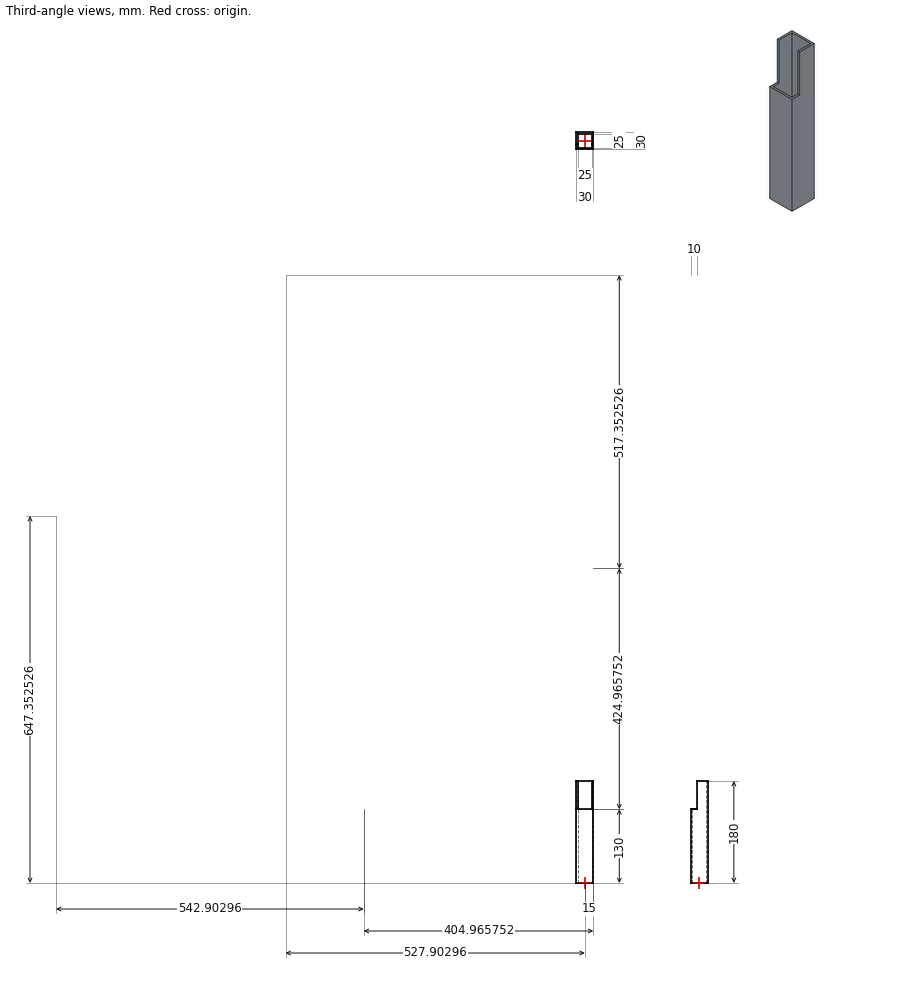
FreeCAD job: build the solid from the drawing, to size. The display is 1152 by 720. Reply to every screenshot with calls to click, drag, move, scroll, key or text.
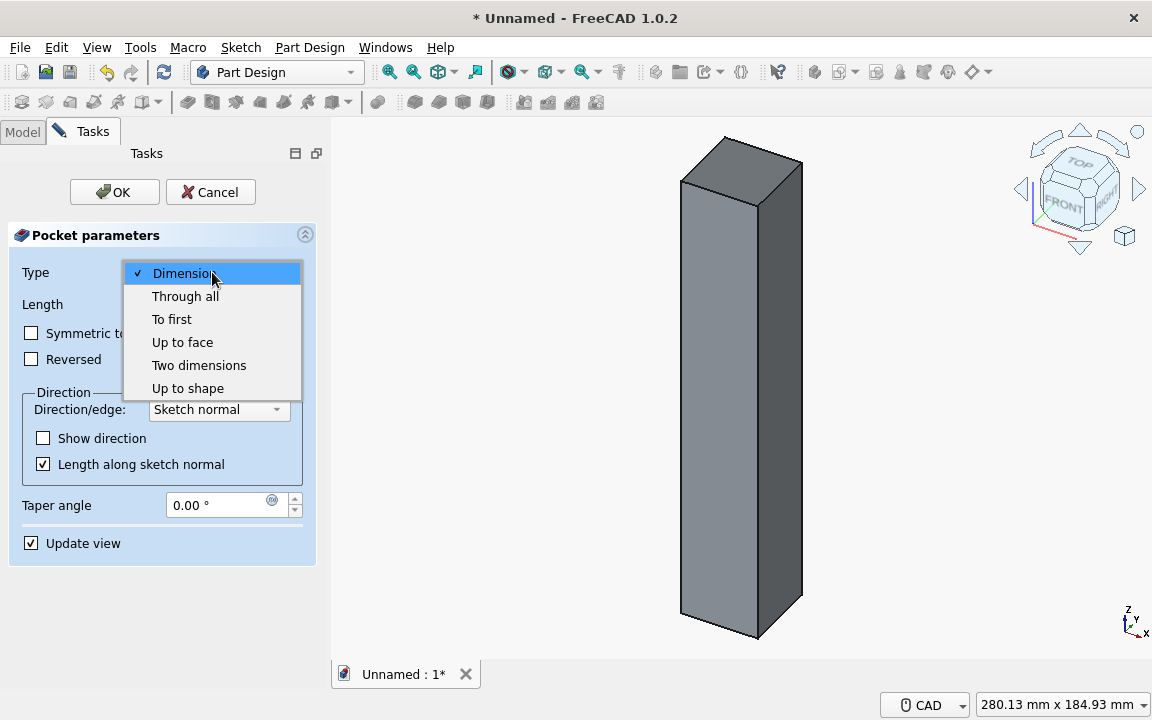
click(212, 296)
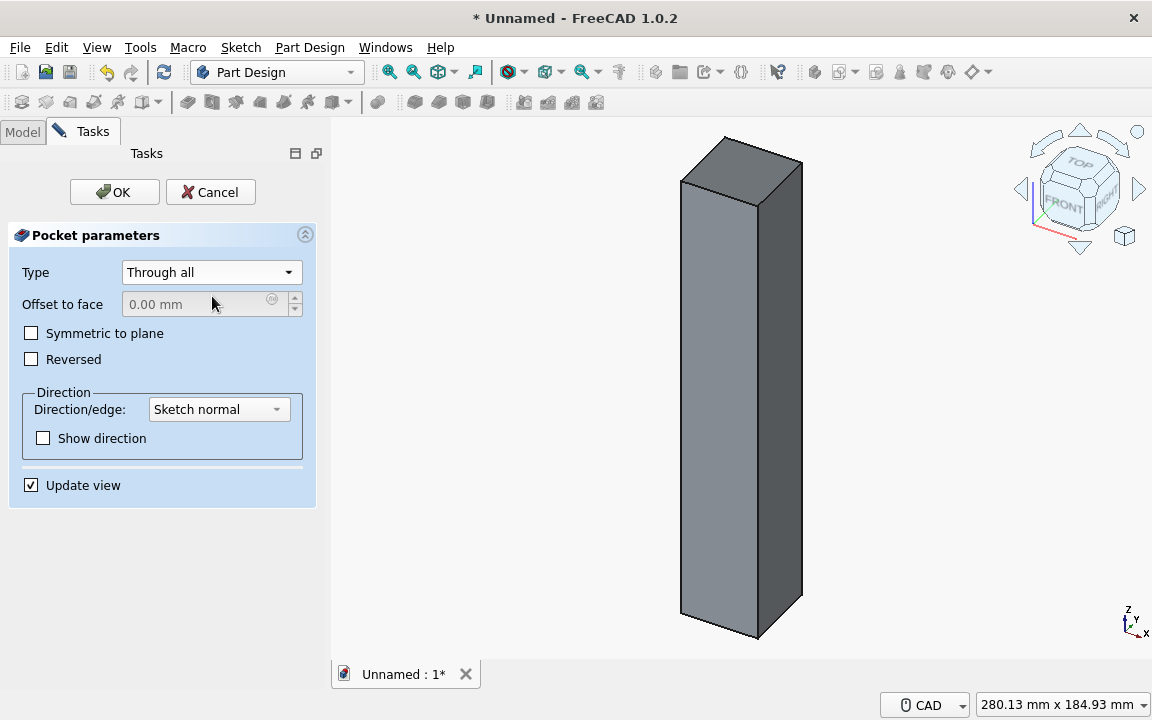
click(30, 359)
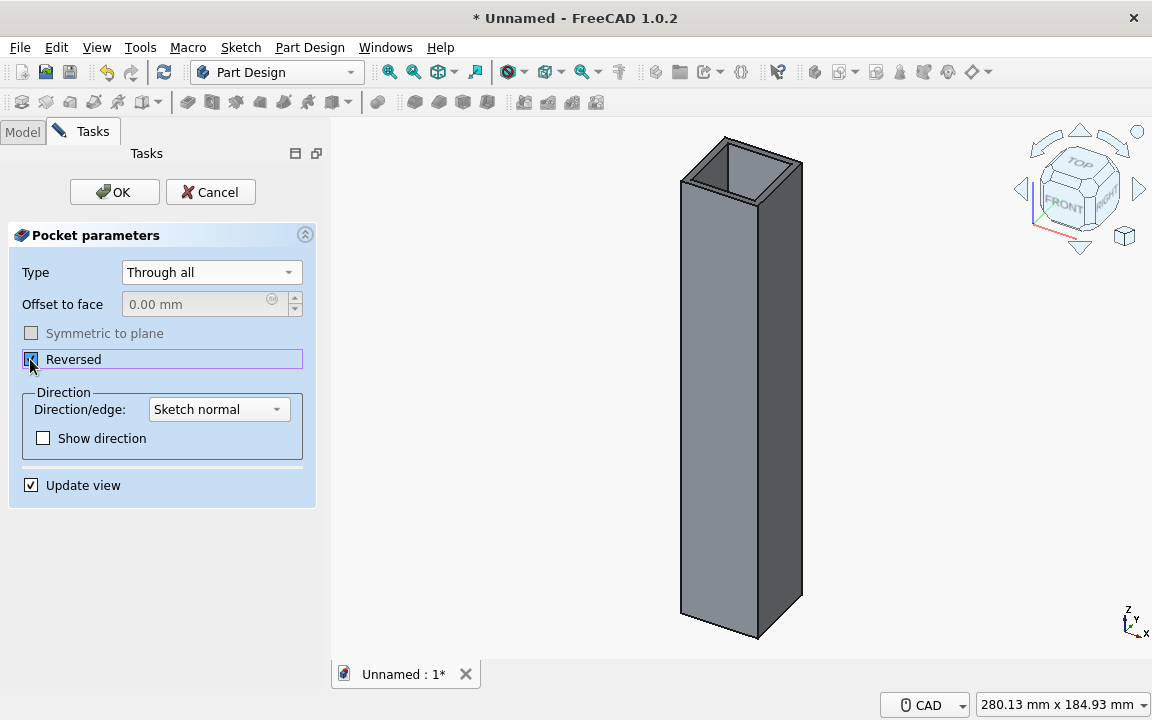
click(115, 192)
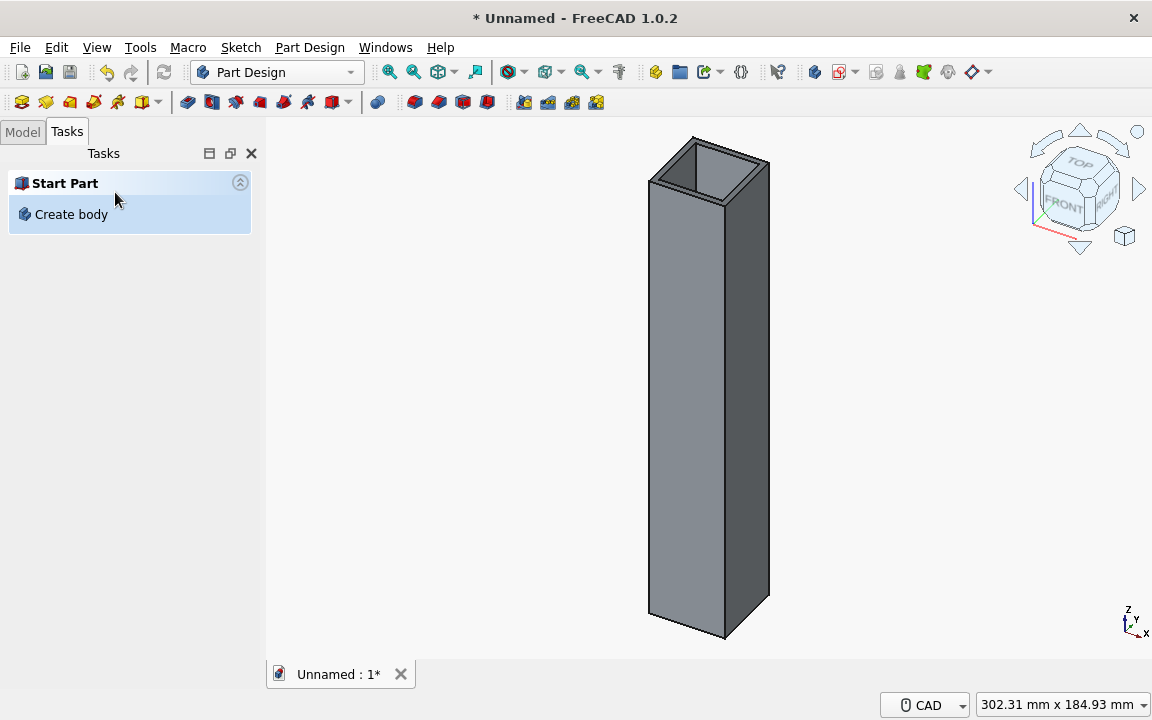
click(687, 285)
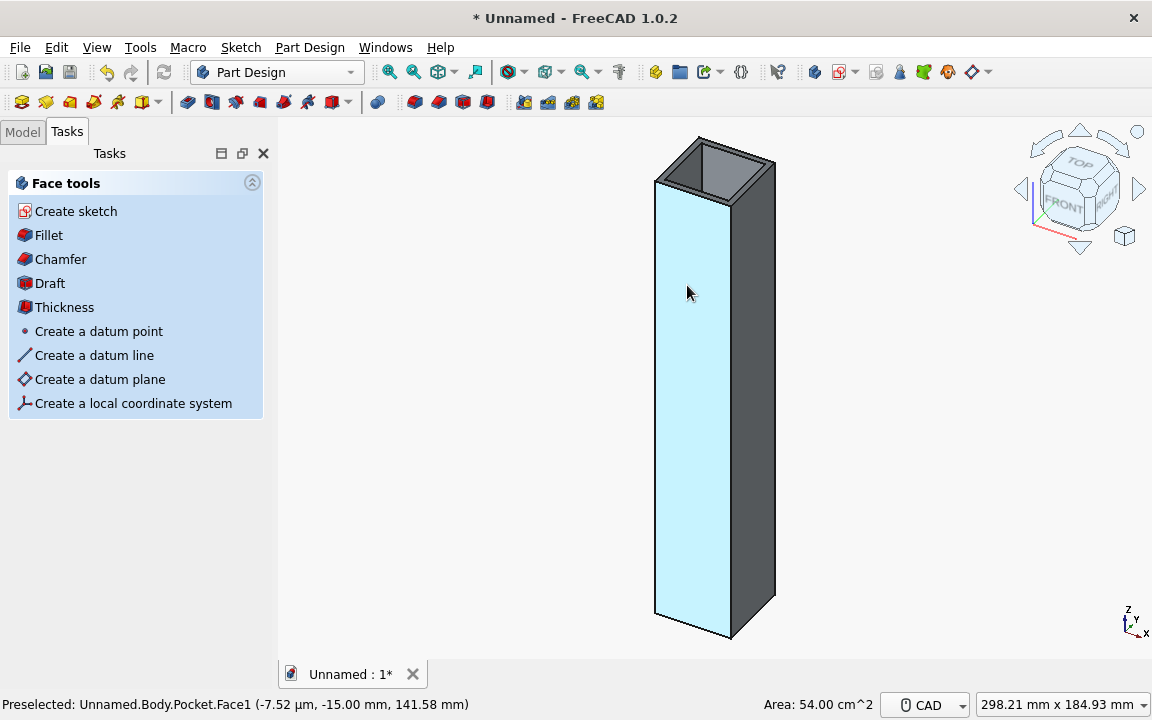
click(840, 72)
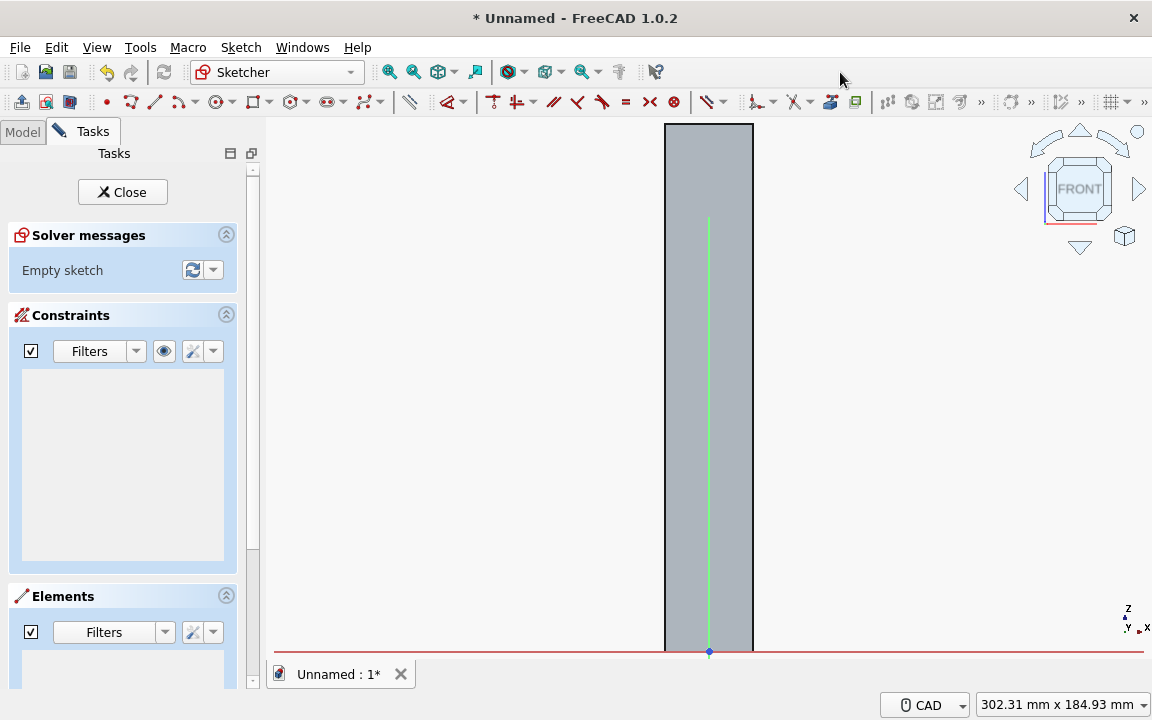
scroll(800, 551, down, 11)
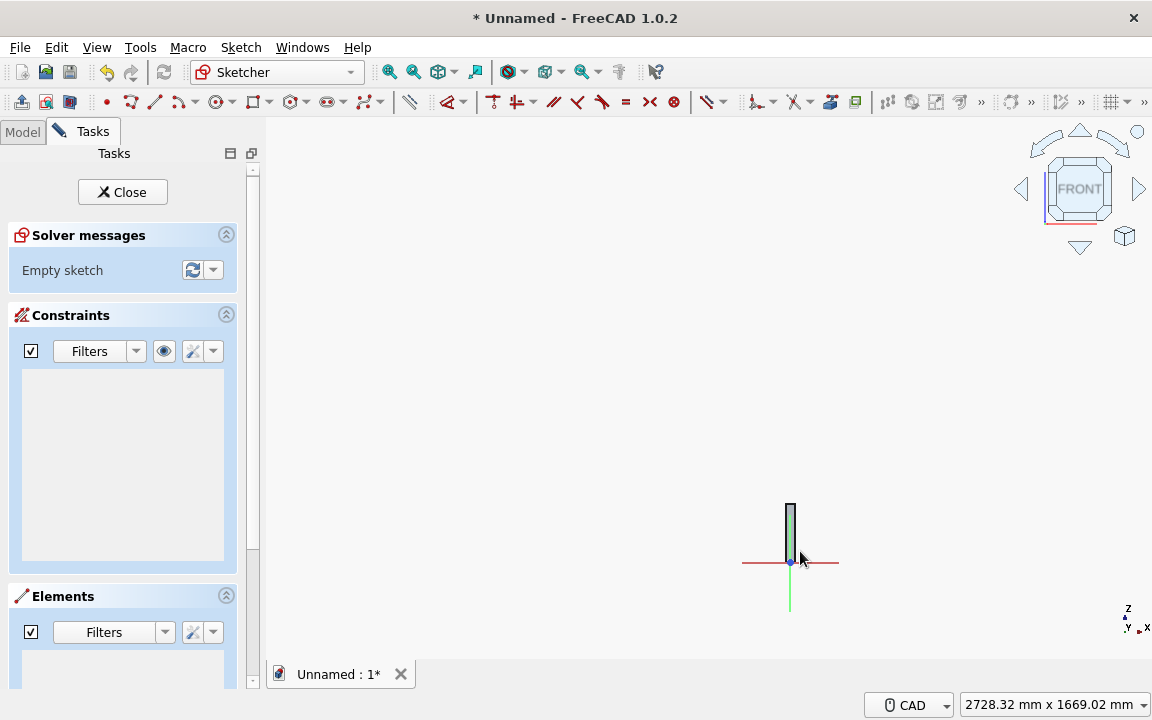
key(g)
key(m)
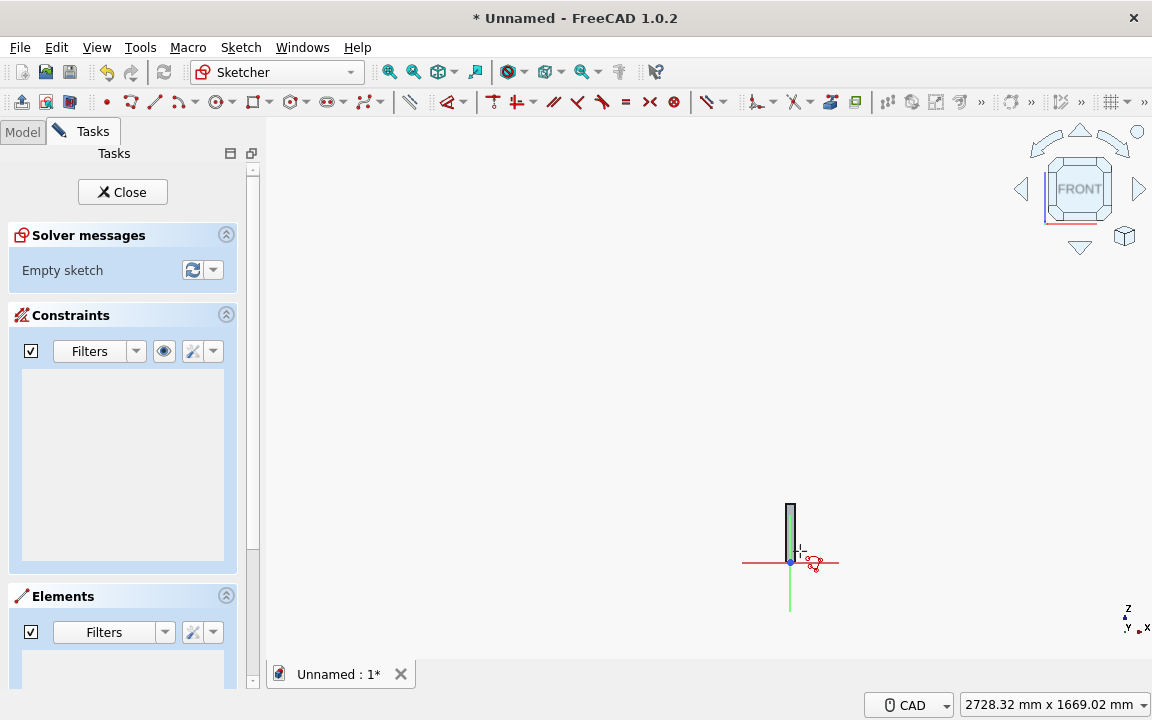
scroll(795, 521, up, 6)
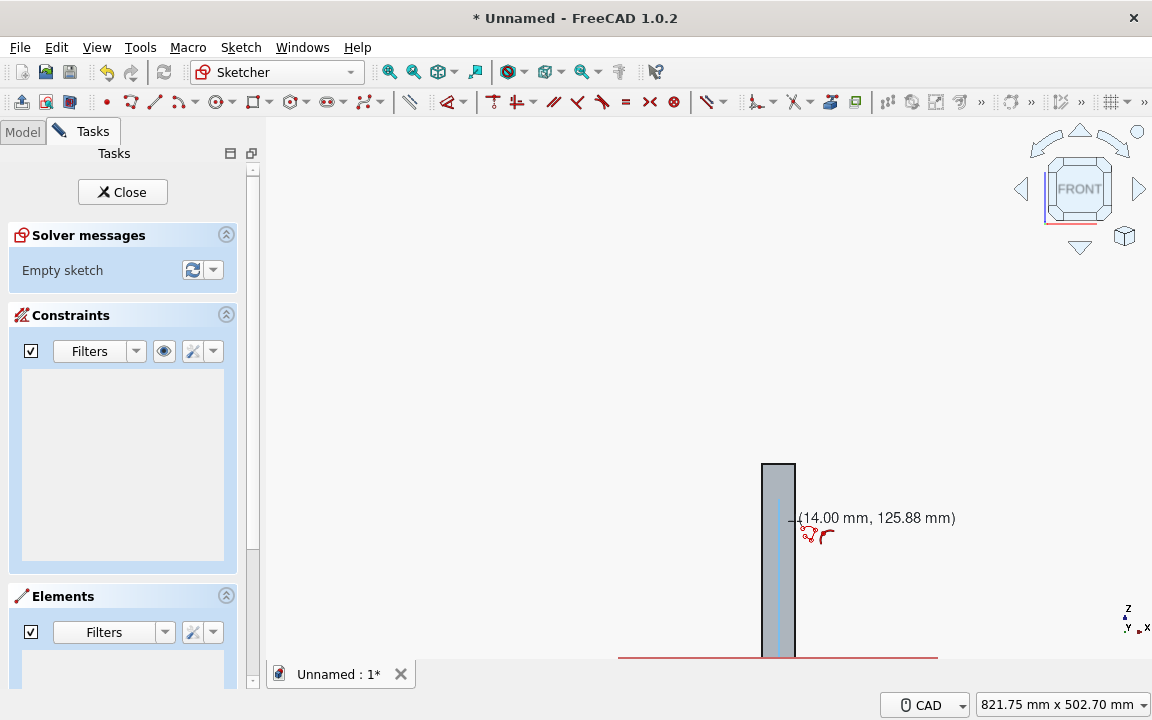
click(795, 518)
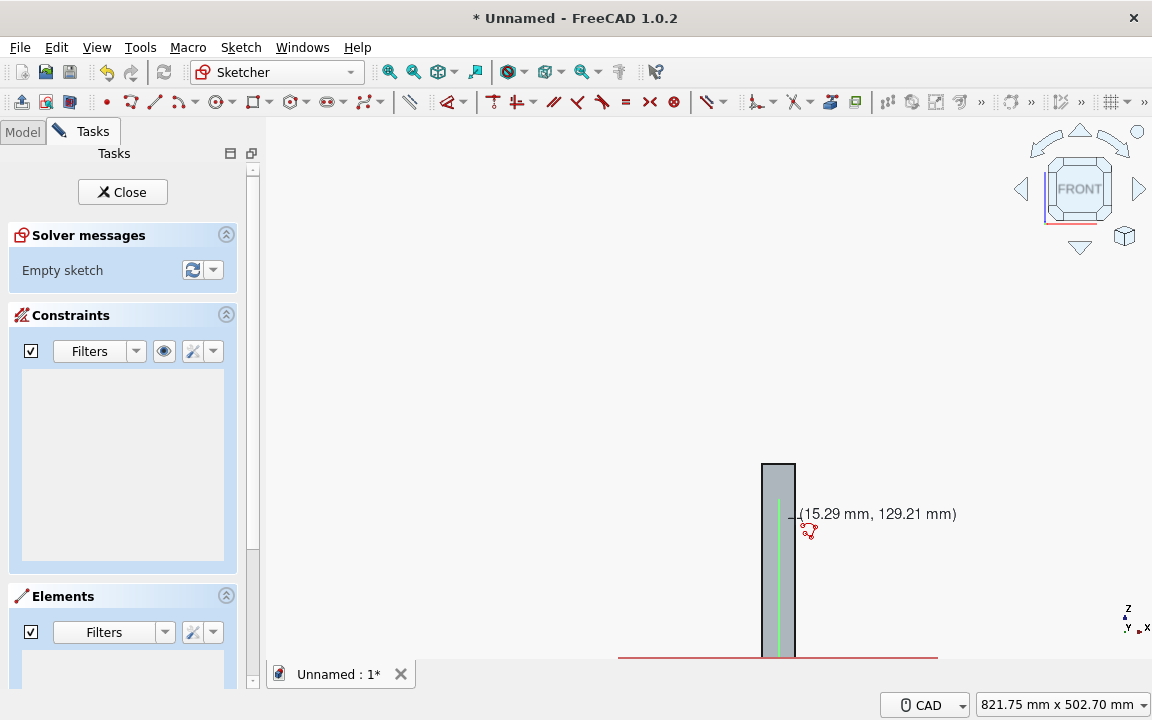
scroll(794, 521, down, 6)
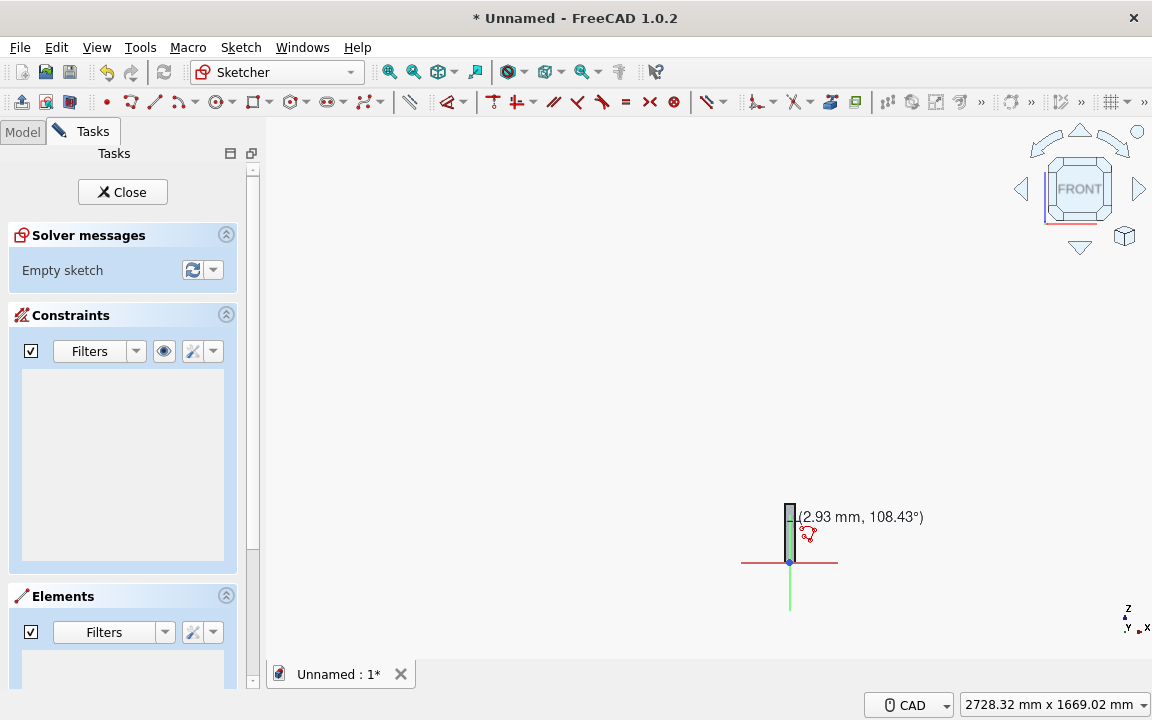
scroll(795, 383, up, 6)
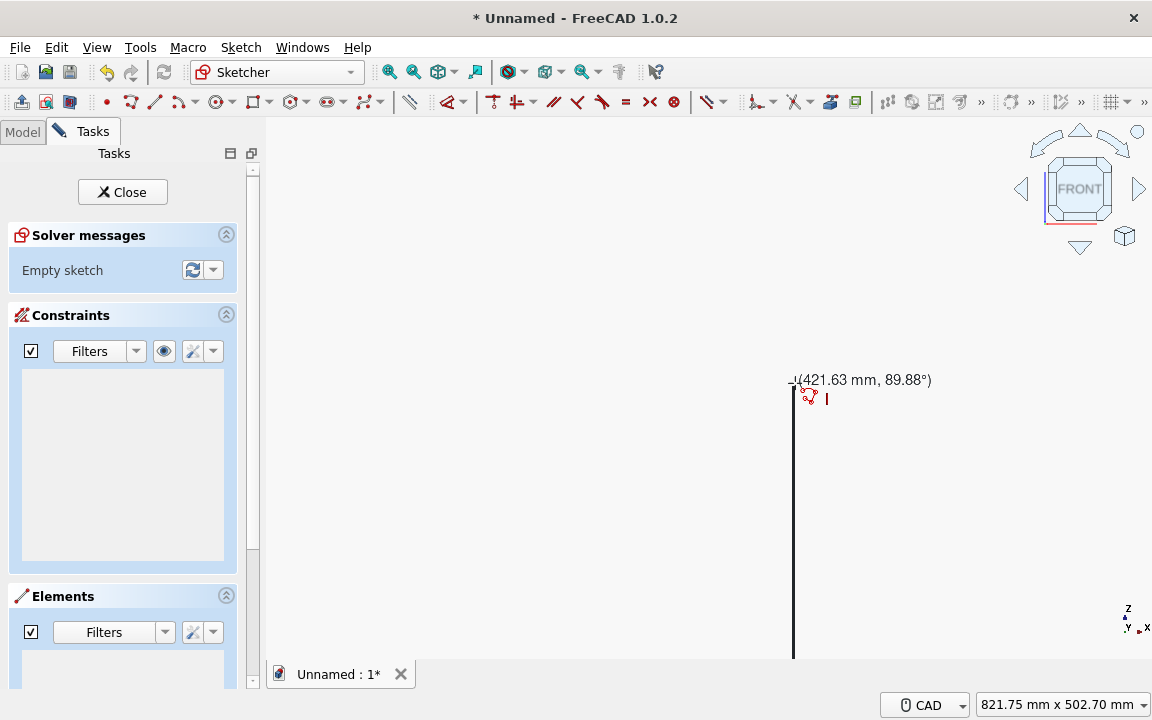
click(793, 381)